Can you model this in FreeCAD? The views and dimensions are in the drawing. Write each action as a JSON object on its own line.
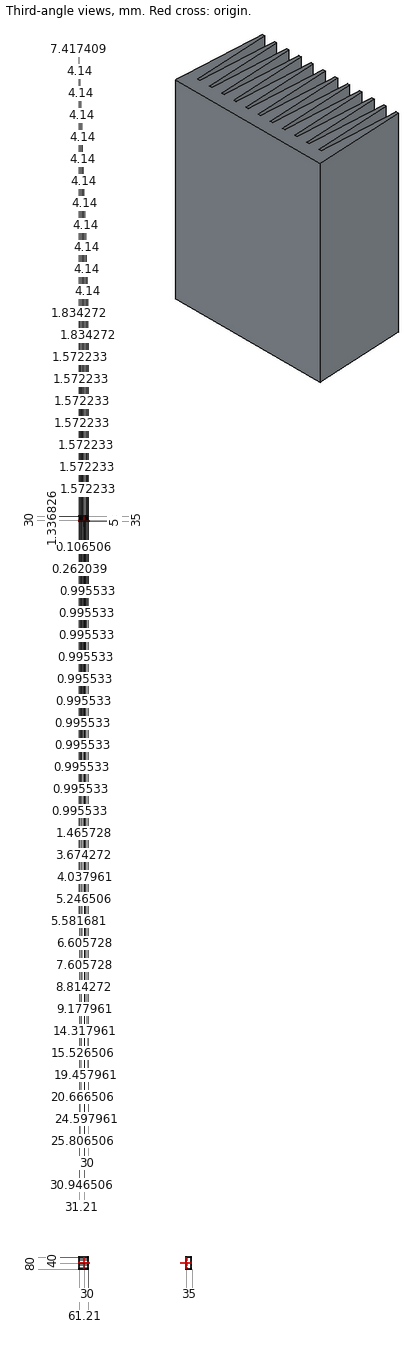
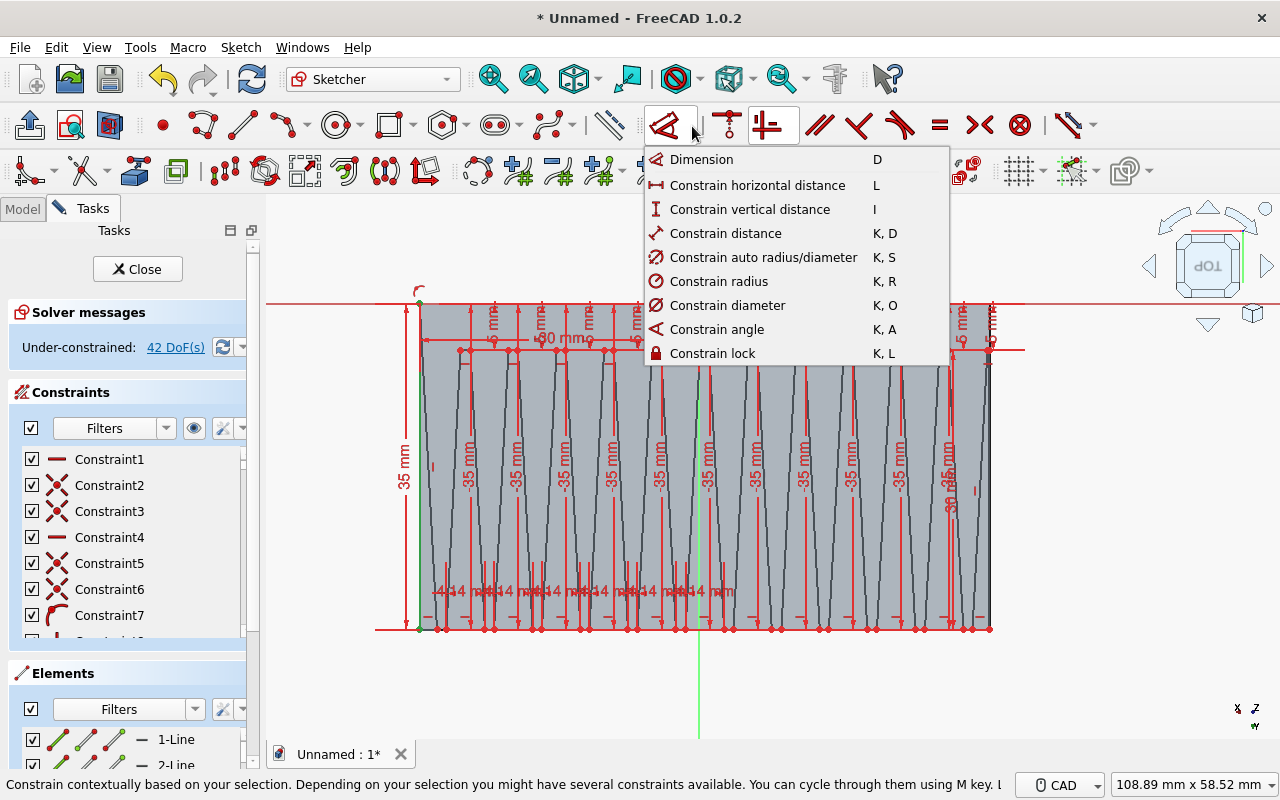
{"action": "left_click", "coordinate": [797, 185]}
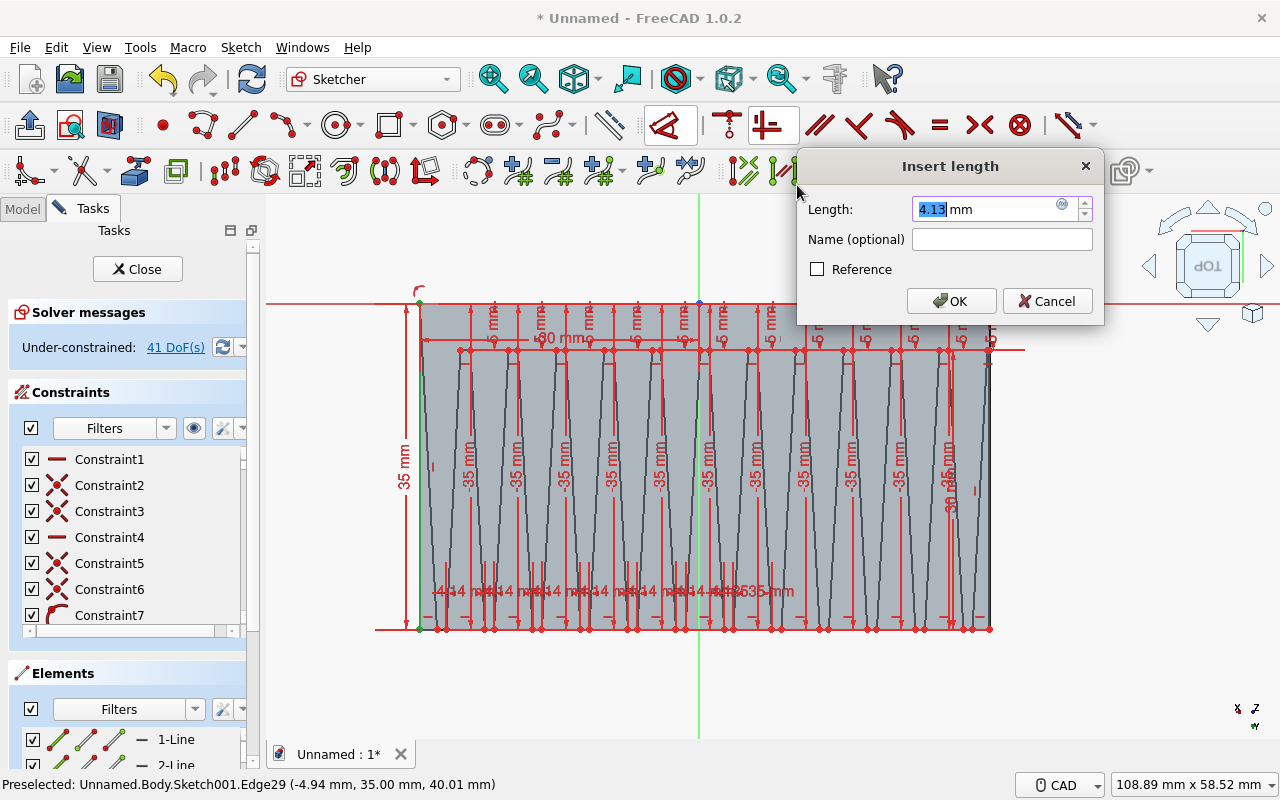
{"action": "type", "text": "4.14"}
{"action": "key", "text": "Return"}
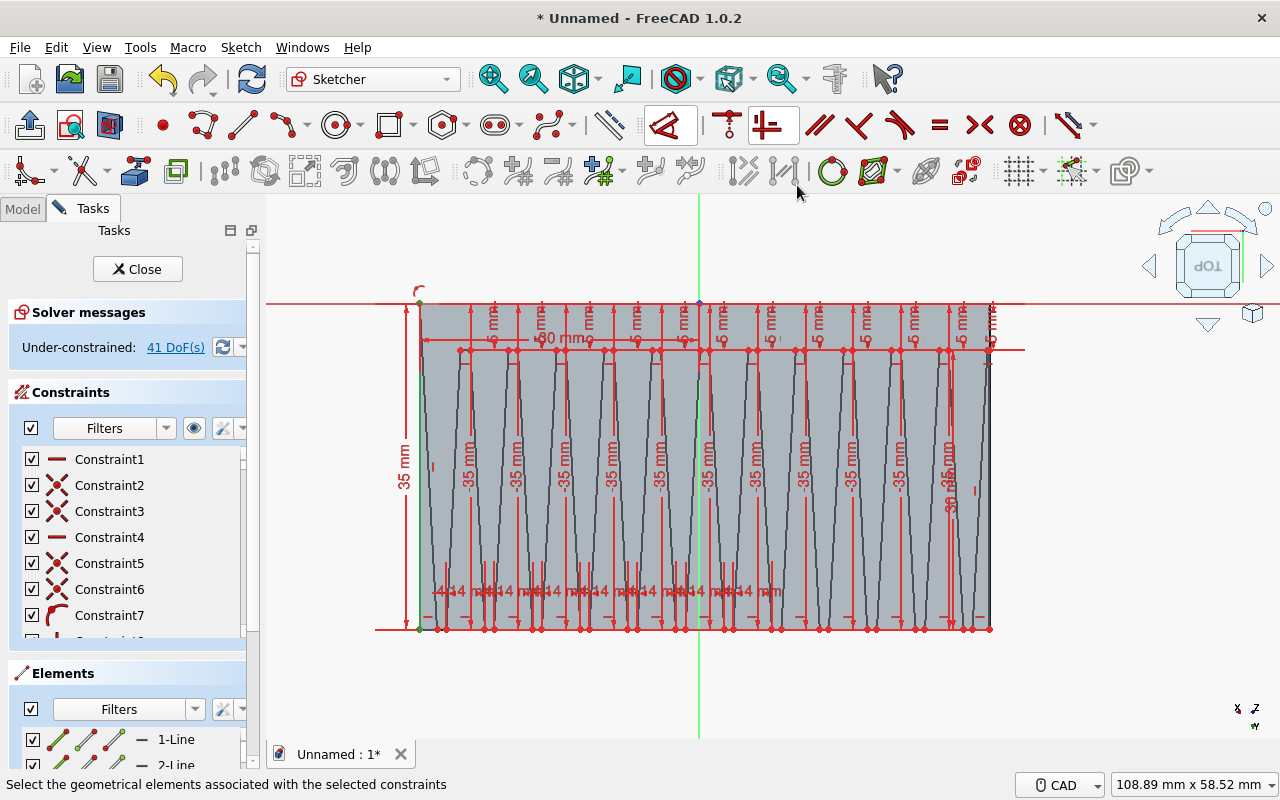
{"action": "left_click", "coordinate": [793, 630]}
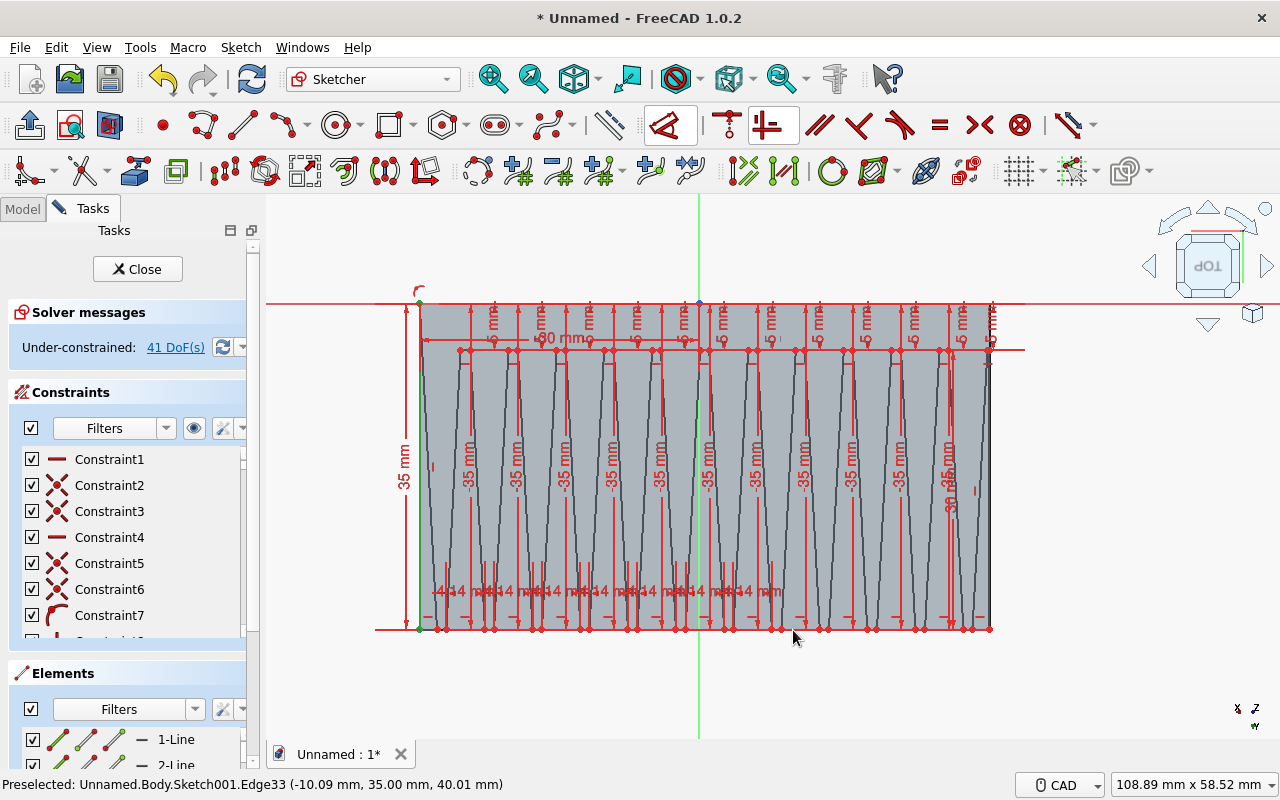
{"action": "key", "text": "l"}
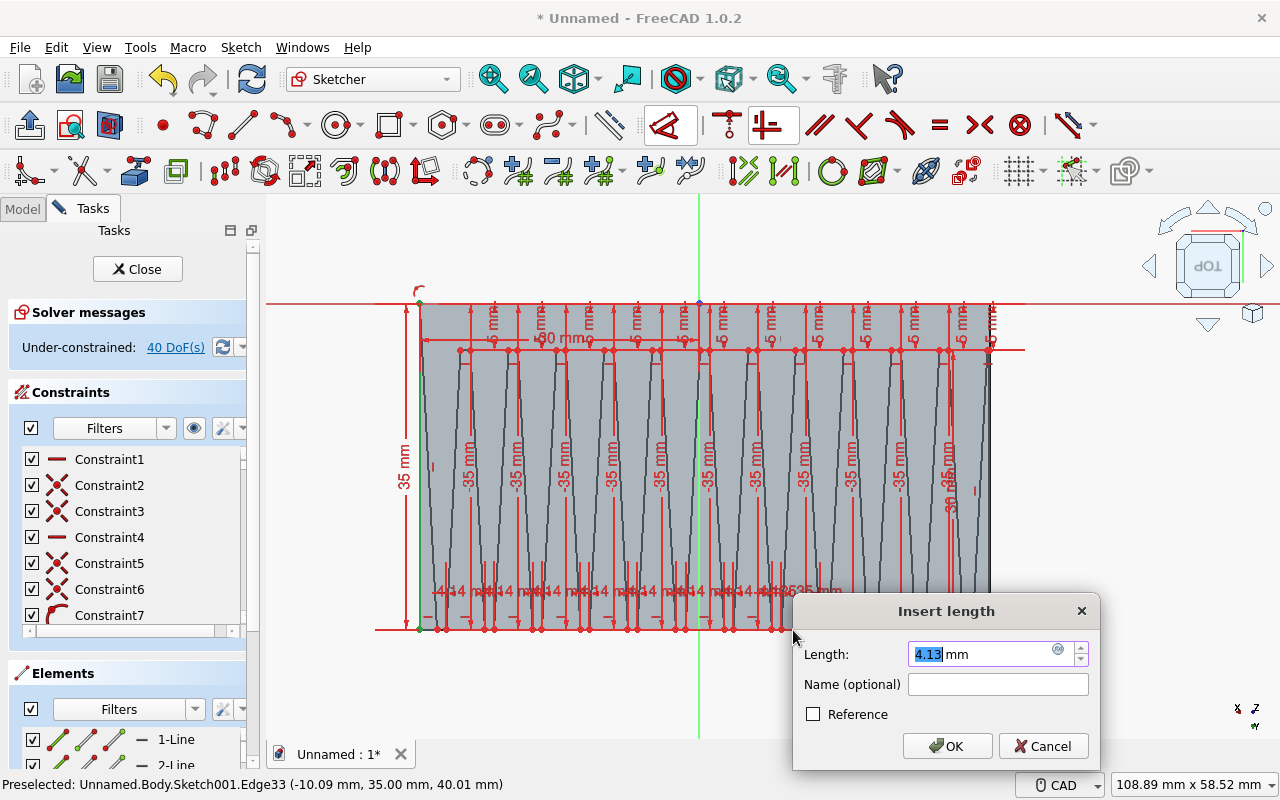
{"action": "type", "text": "4.14"}
{"action": "key", "text": "Return"}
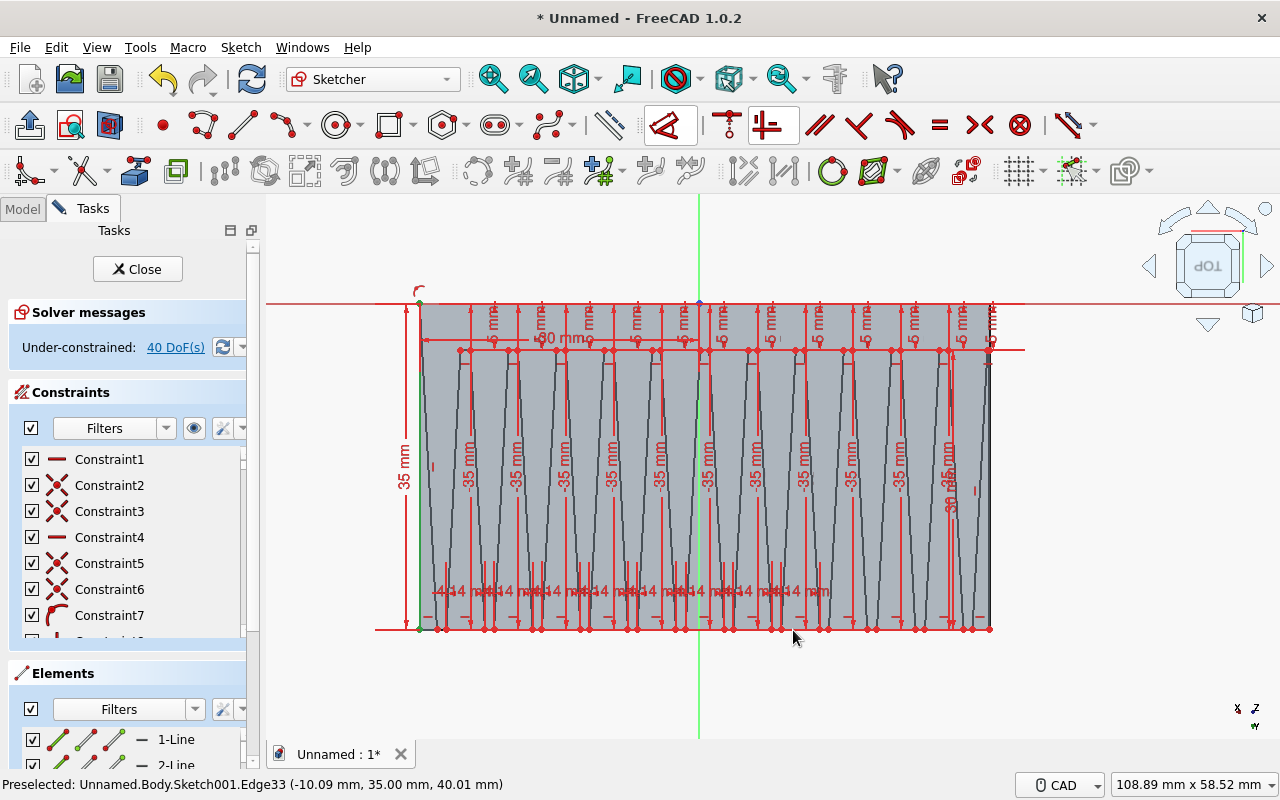
{"action": "left_click", "coordinate": [840, 630]}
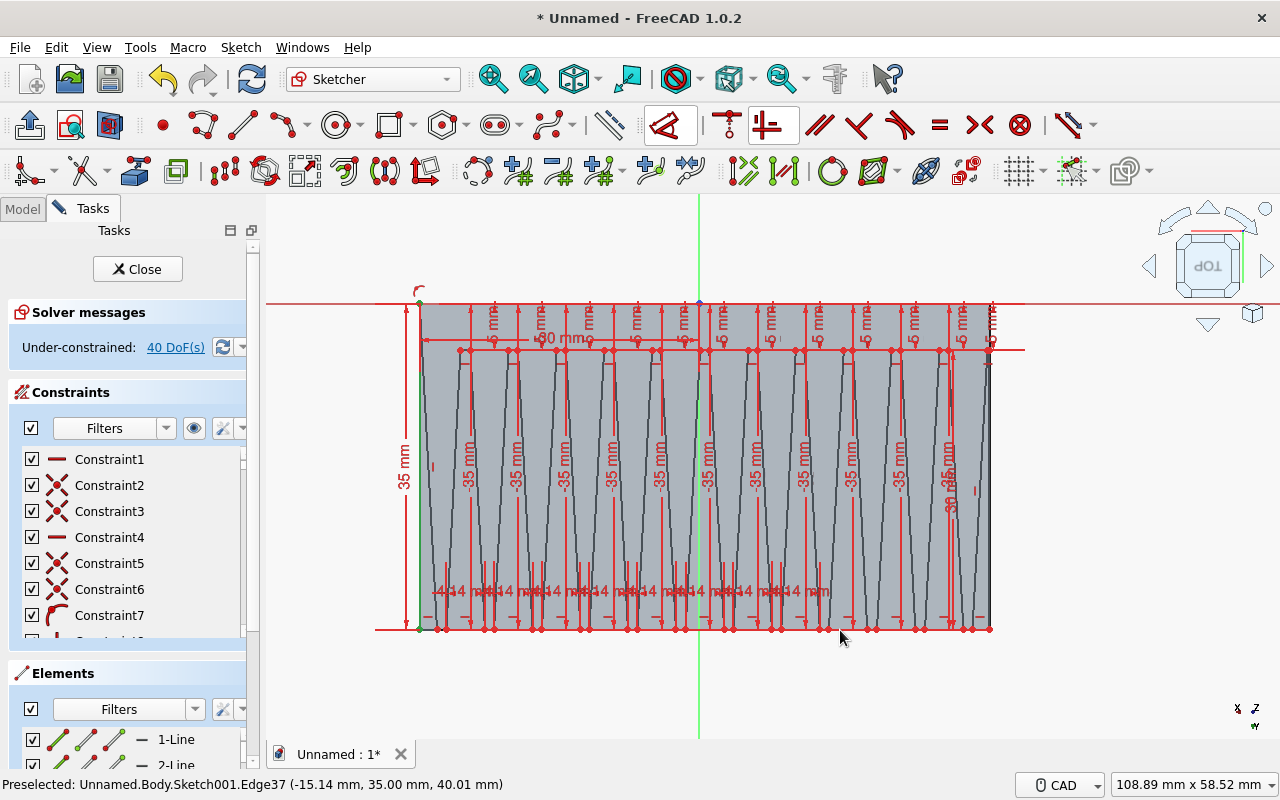
{"action": "key", "text": "l"}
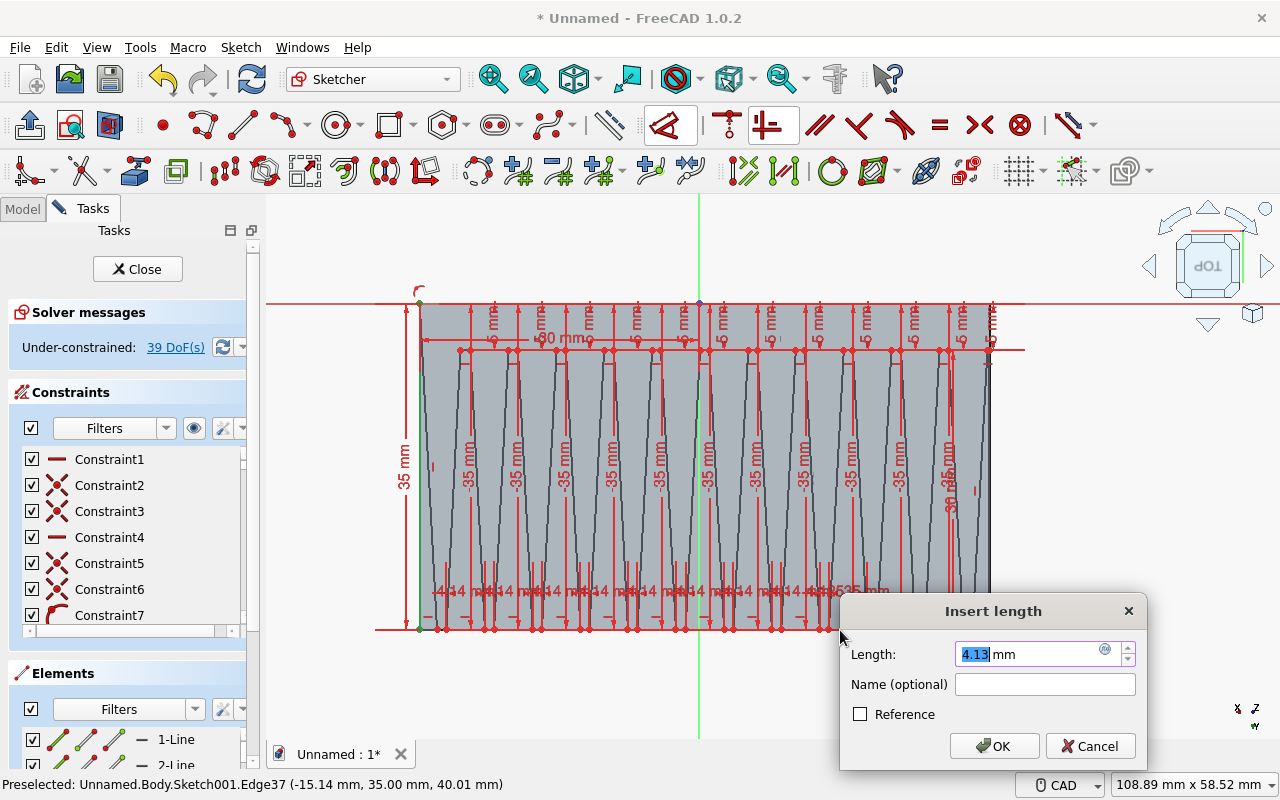
{"action": "type", "text": "4.14"}
{"action": "key", "text": "Return"}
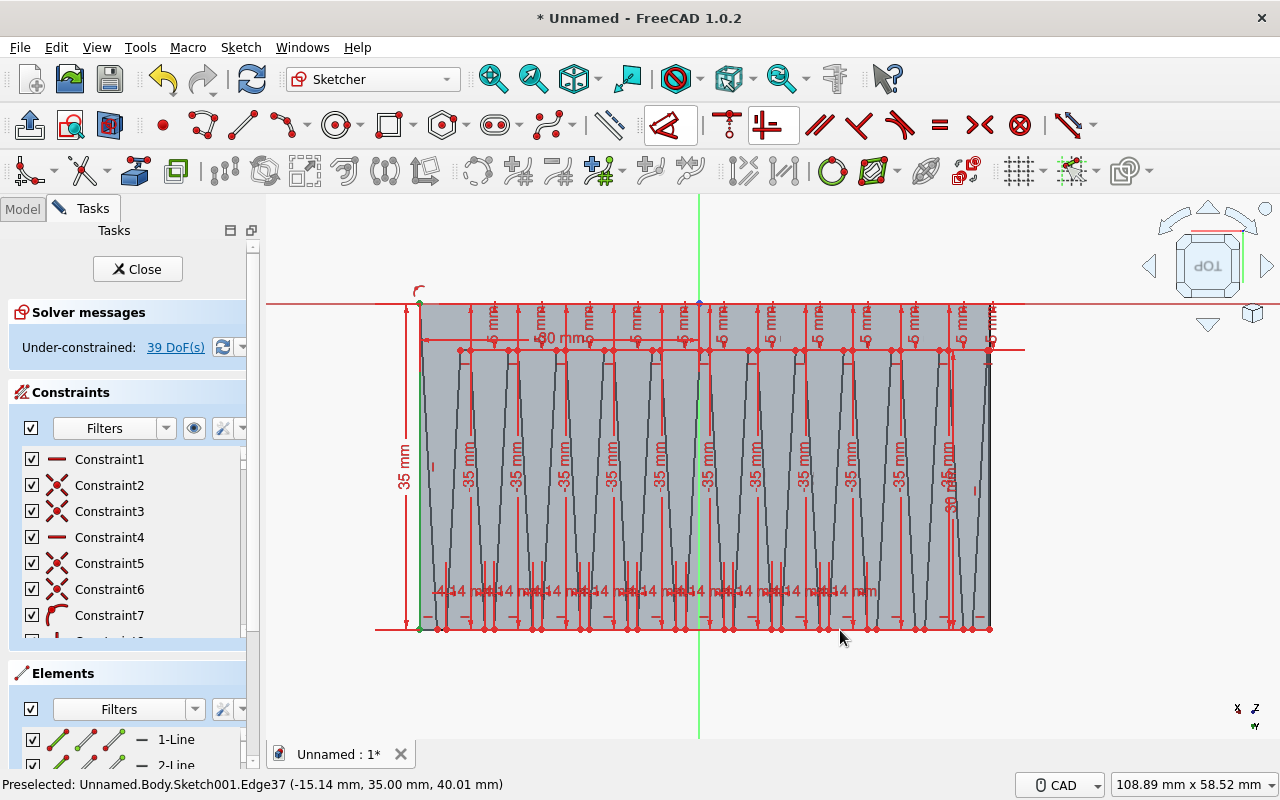
{"action": "left_click", "coordinate": [888, 630]}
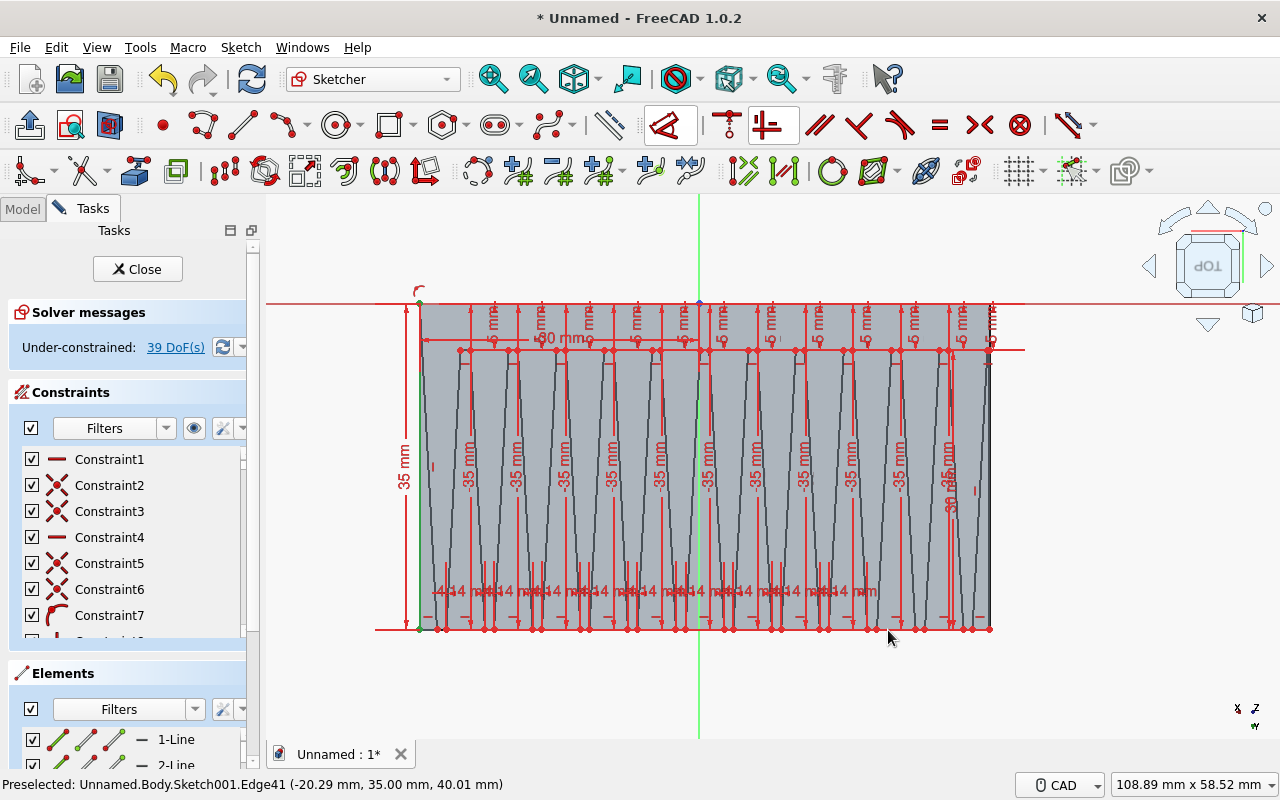
{"action": "key", "text": "l"}